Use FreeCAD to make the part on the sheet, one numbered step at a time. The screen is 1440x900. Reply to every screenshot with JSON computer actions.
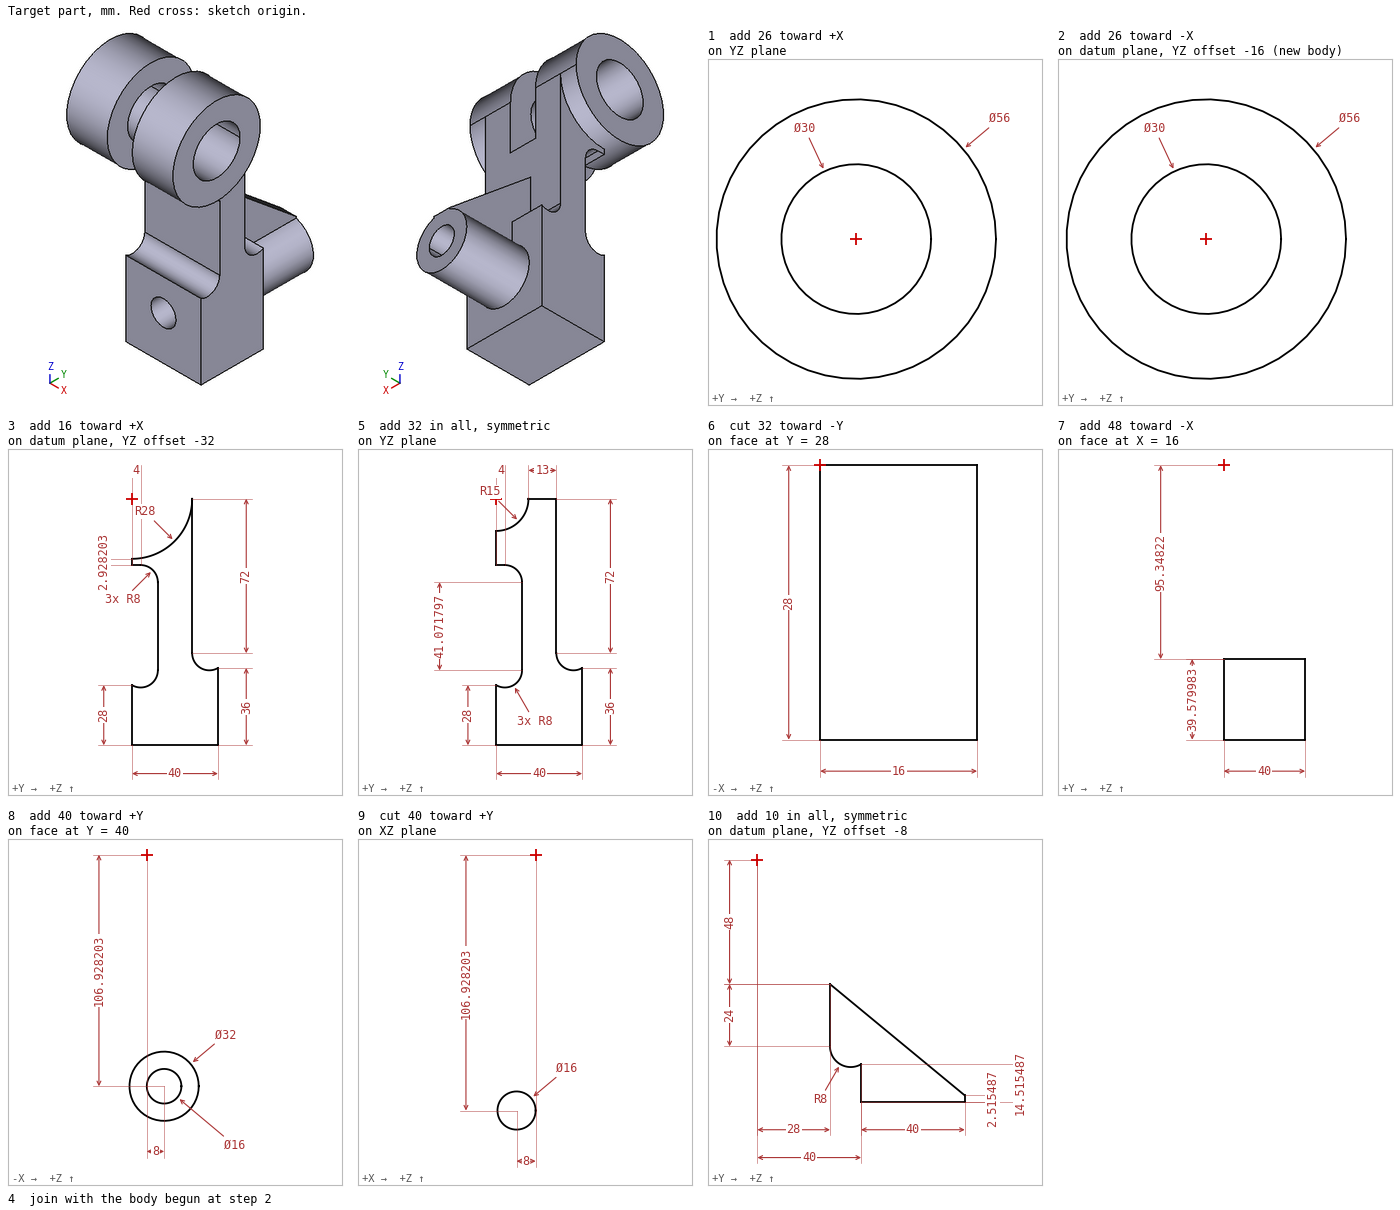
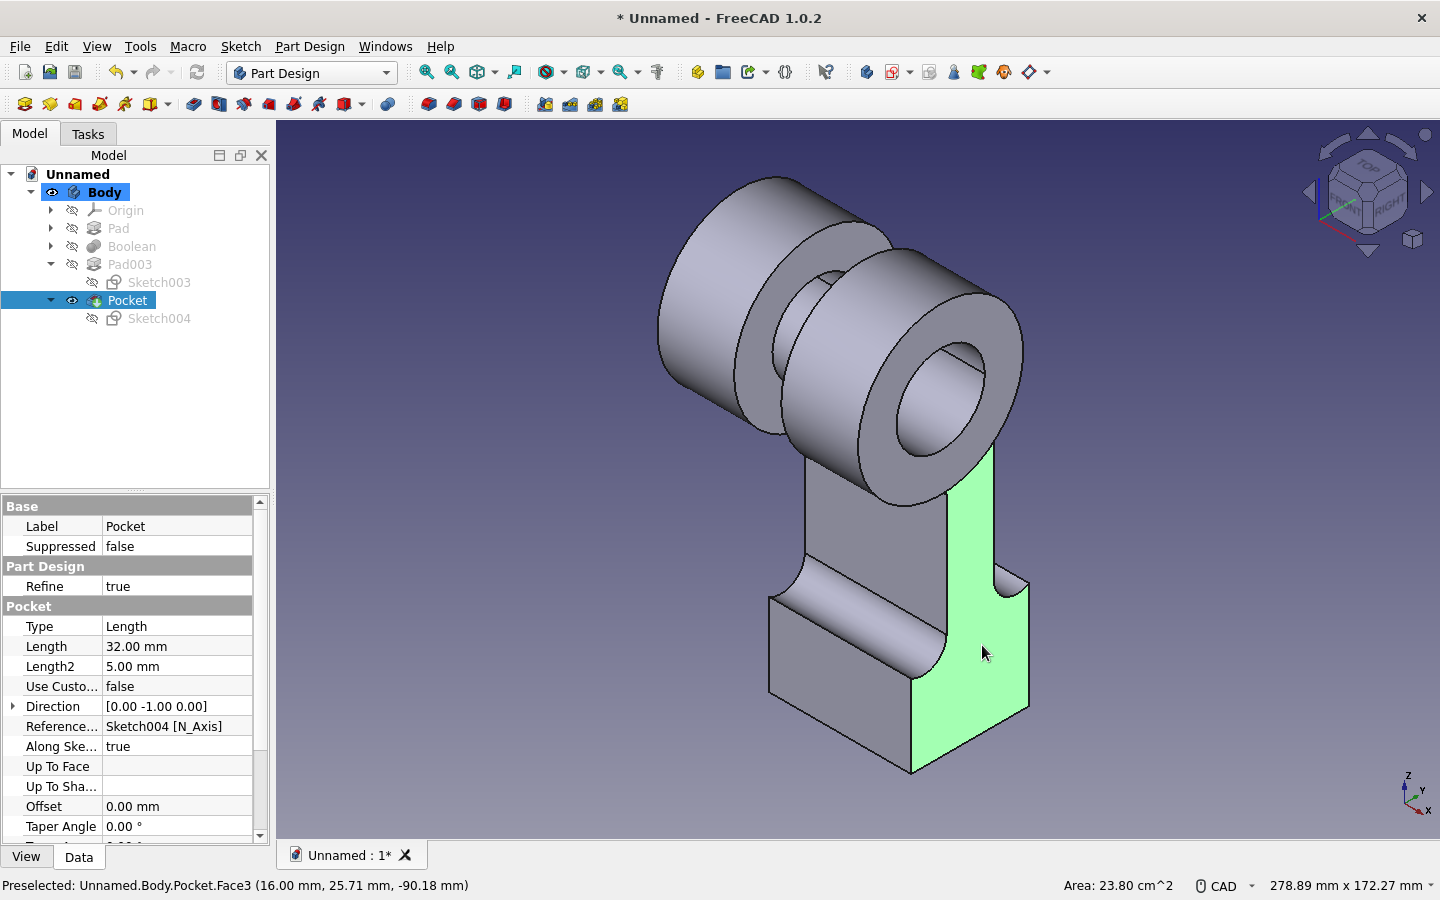
{"action": "left_click", "coordinate": [892, 72]}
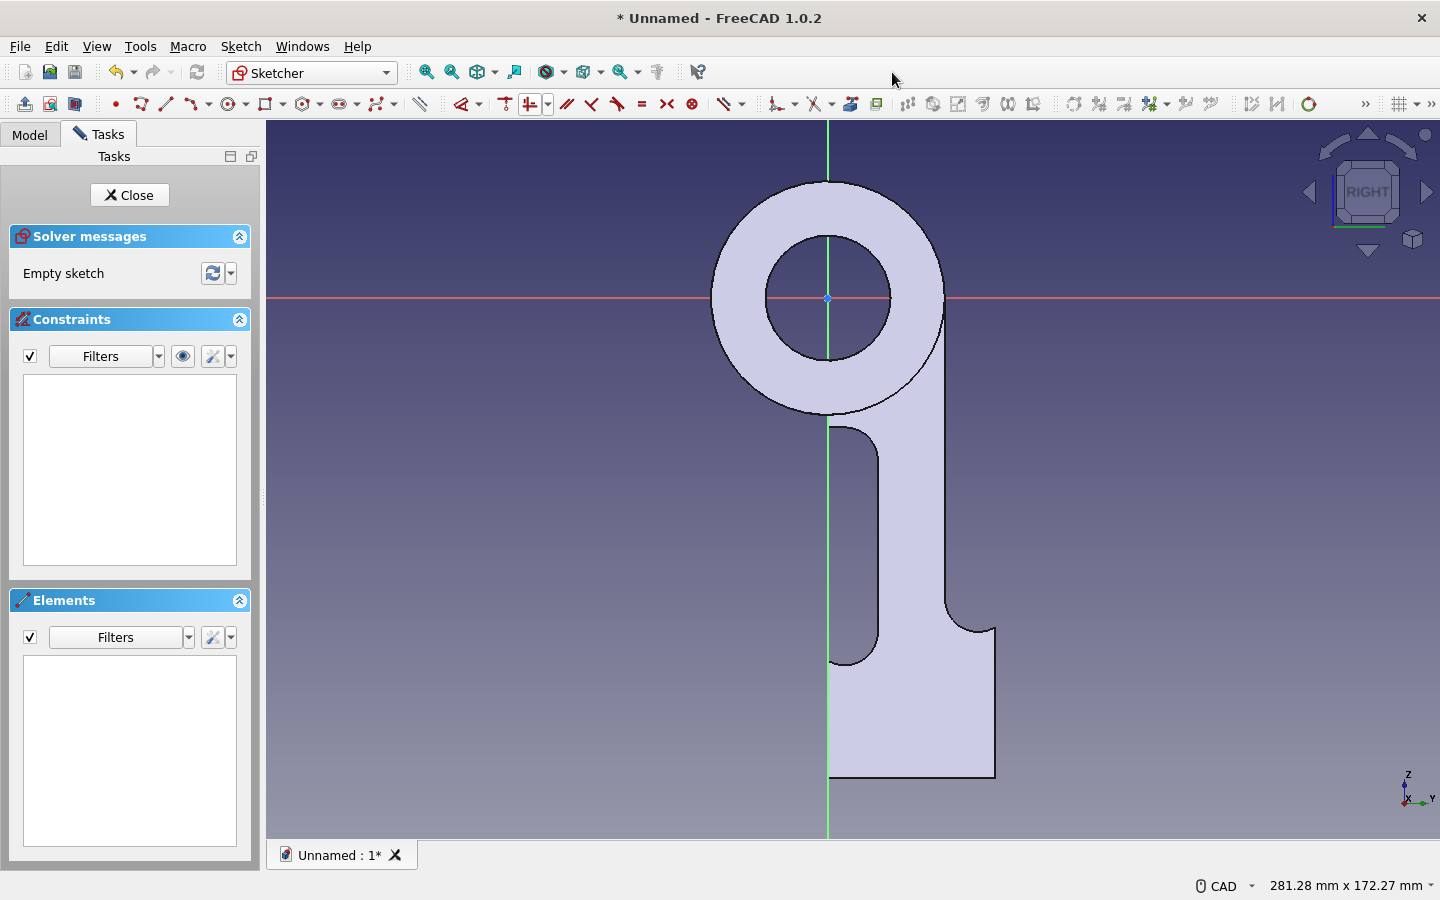
{"action": "scroll", "coordinate": [784, 480], "scroll_direction": "down", "scroll_amount": 5}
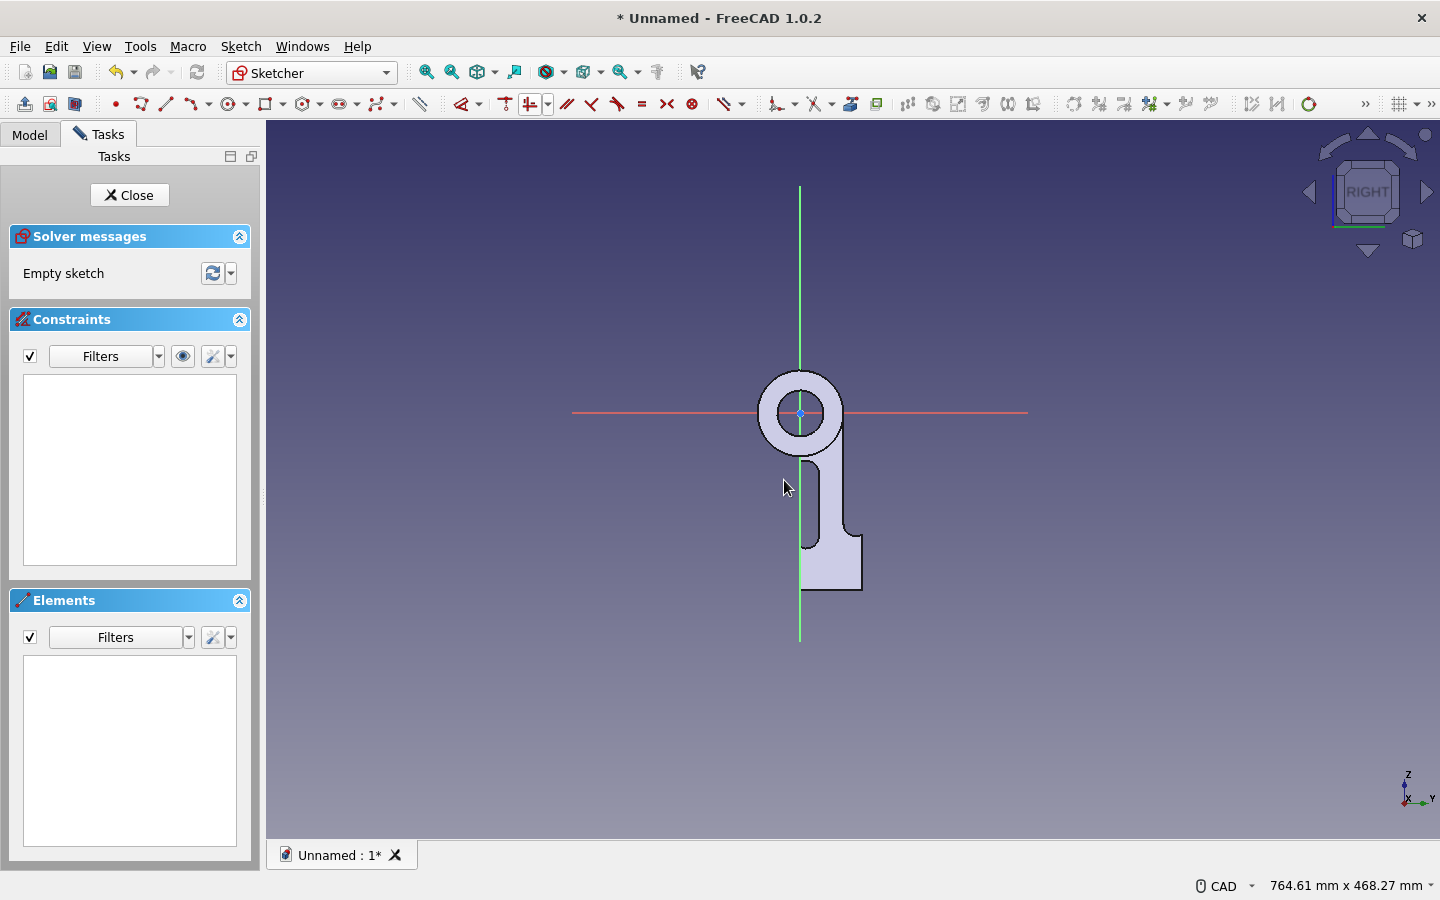
{"action": "scroll", "coordinate": [838, 608], "scroll_direction": "up", "scroll_amount": 10}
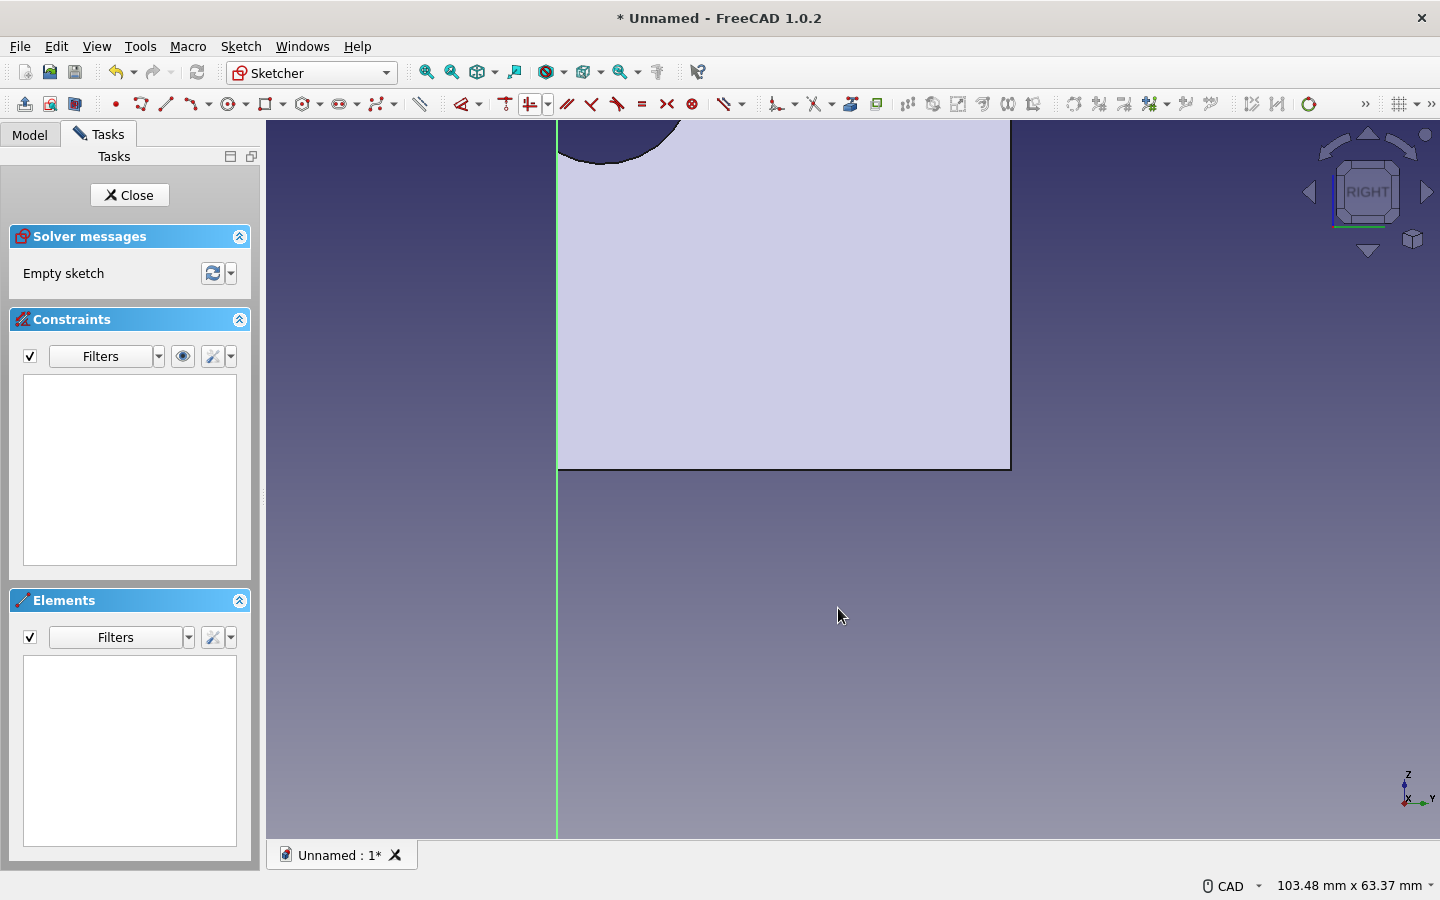
{"action": "left_click", "coordinate": [264, 104]}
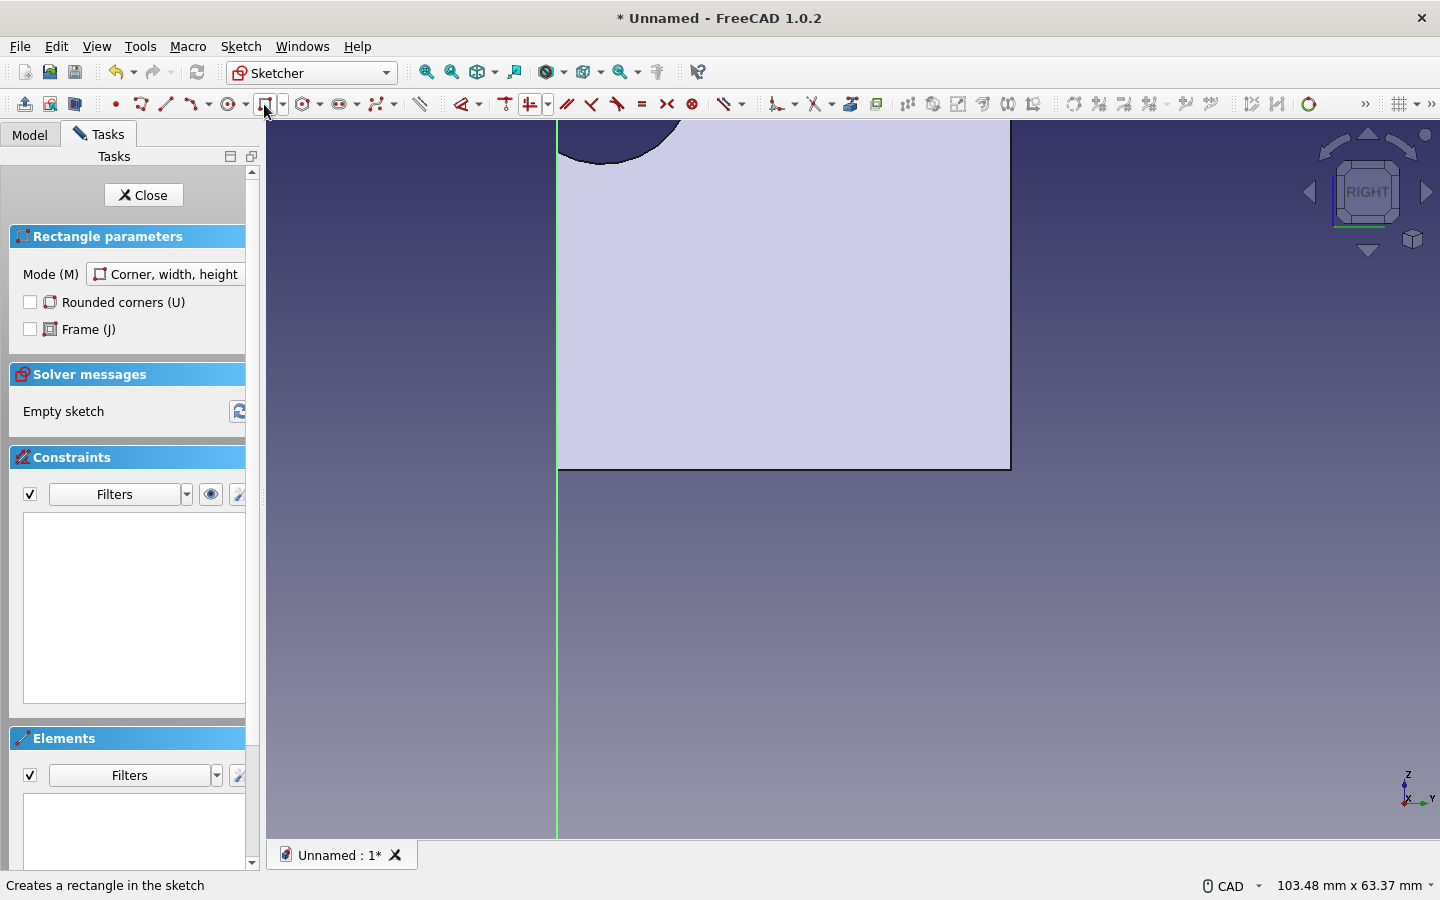
{"action": "left_click", "coordinate": [557, 247]}
{"action": "left_click", "coordinate": [1011, 697]}
{"action": "key", "text": "Escape"}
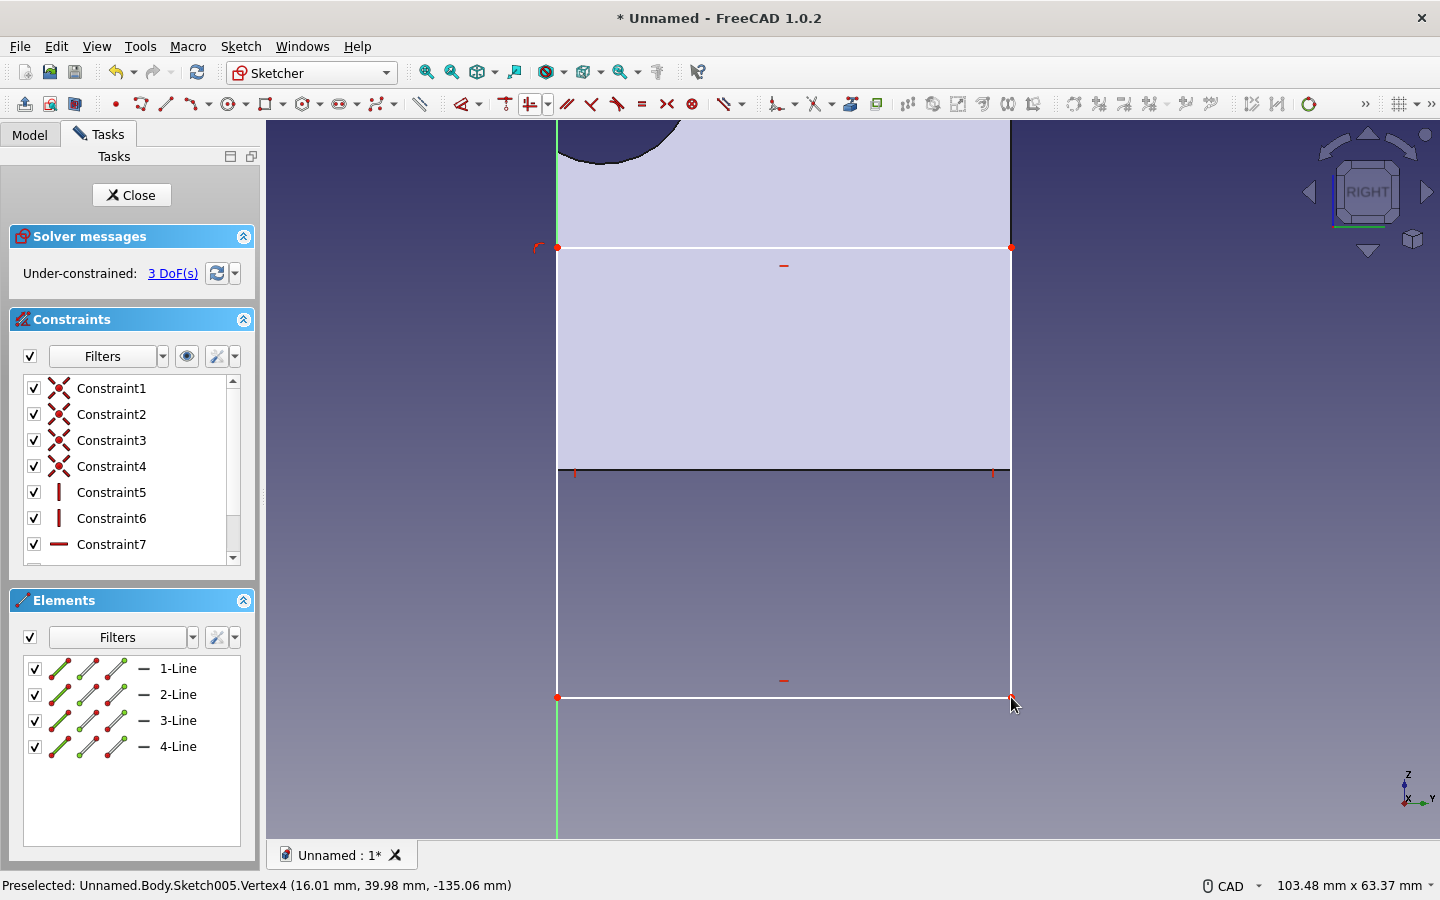
{"action": "left_click", "coordinate": [460, 104]}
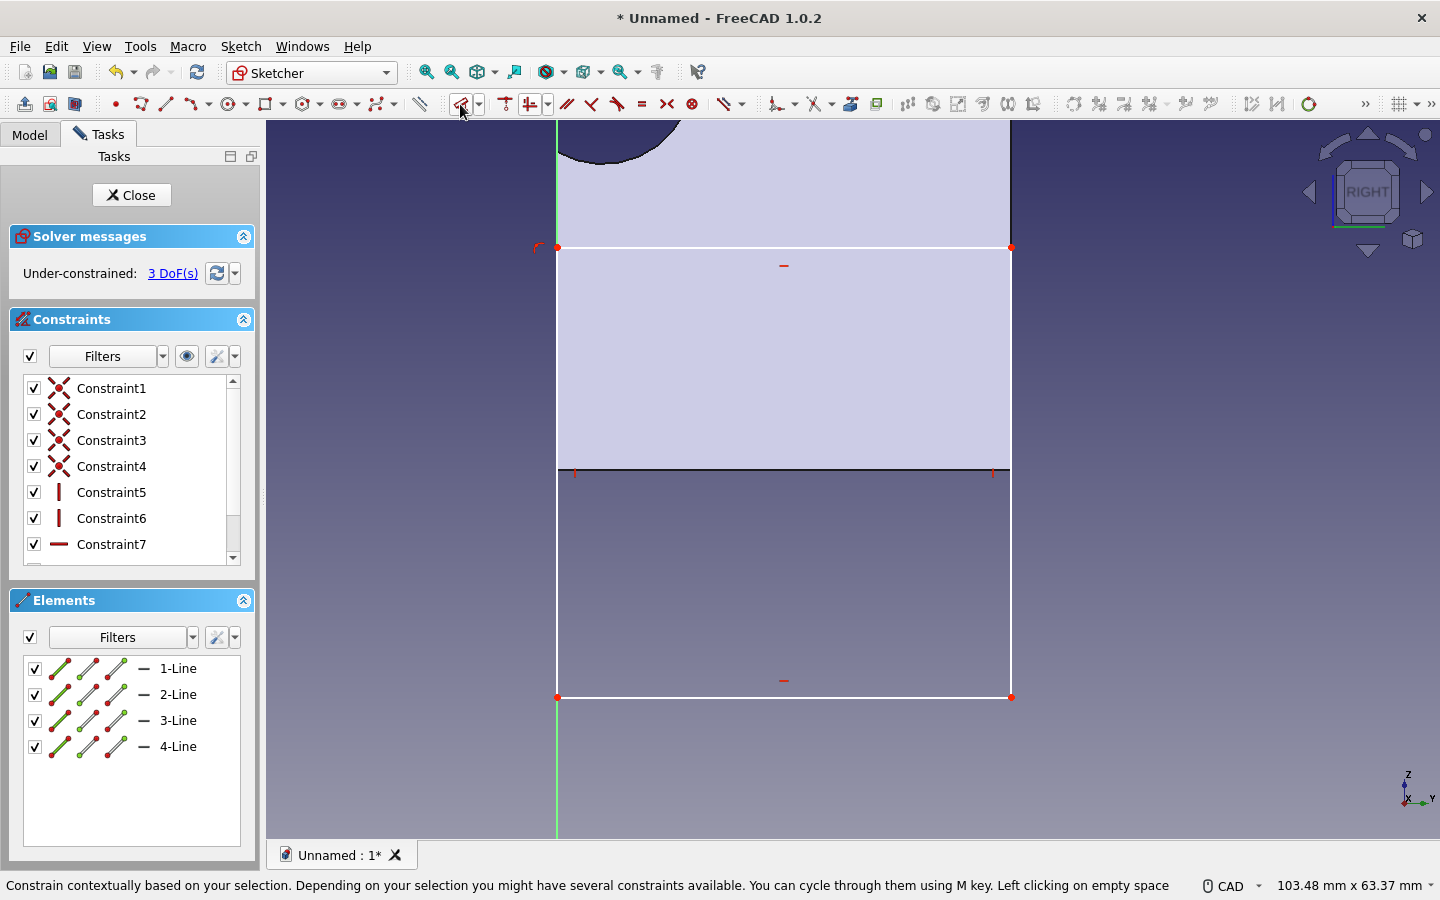
{"action": "left_click", "coordinate": [693, 698]}
{"action": "left_click", "coordinate": [784, 732]}